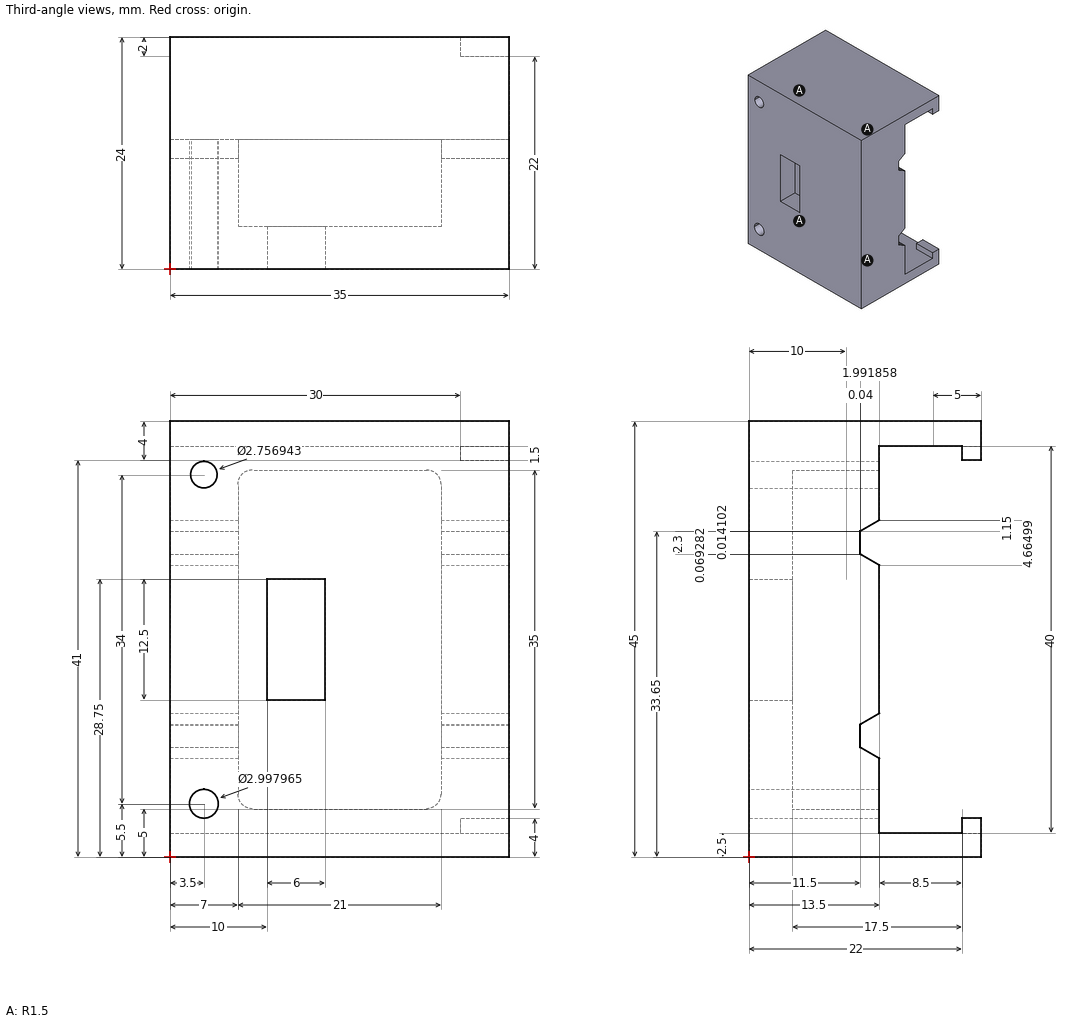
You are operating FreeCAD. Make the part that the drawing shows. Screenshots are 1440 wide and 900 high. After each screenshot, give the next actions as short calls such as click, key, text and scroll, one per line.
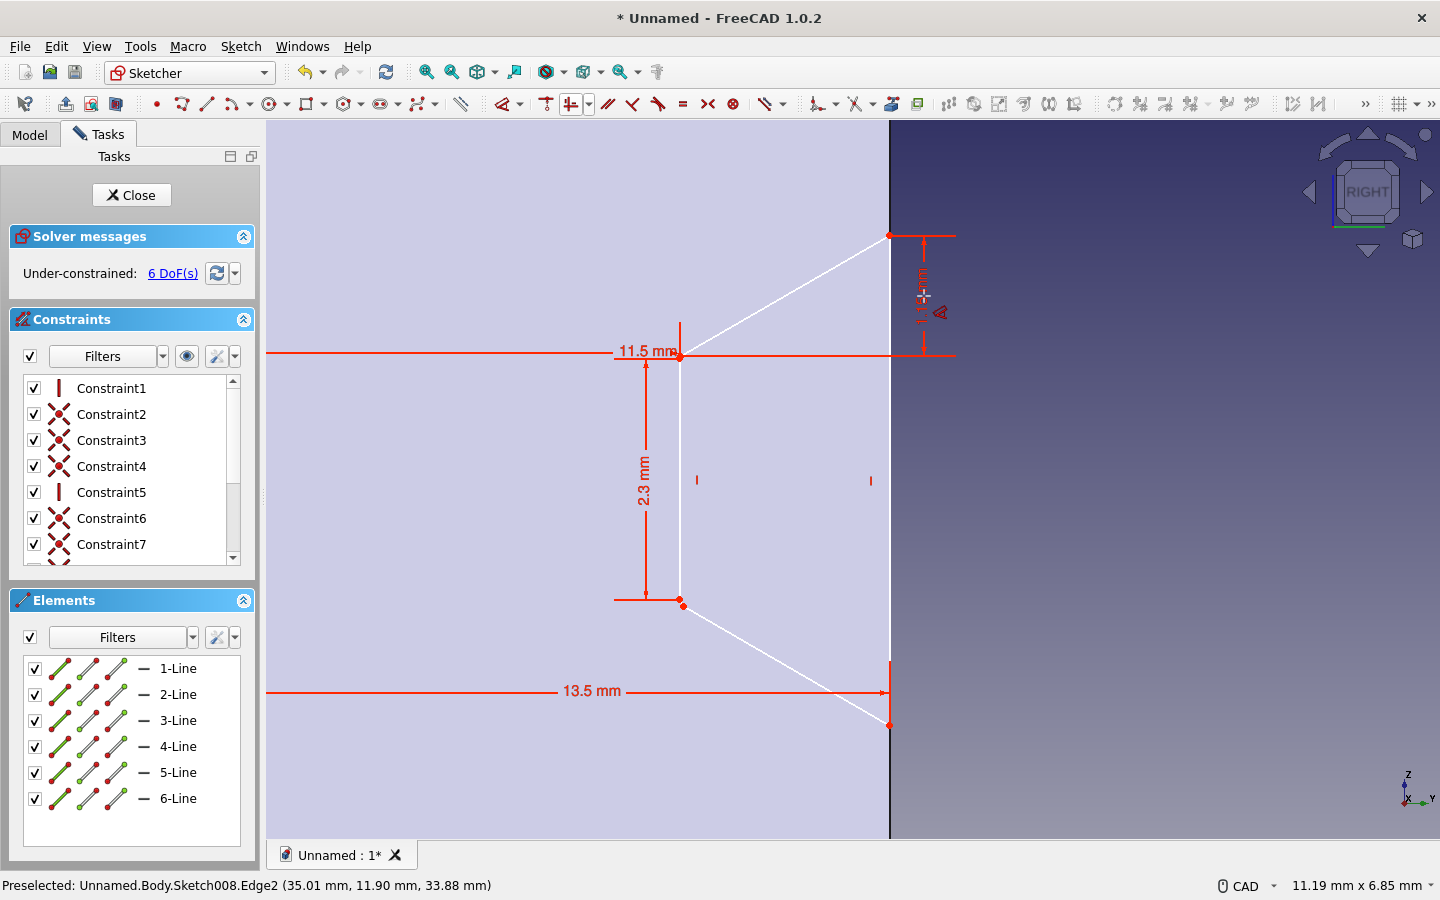
scroll(682, 603, up, 12)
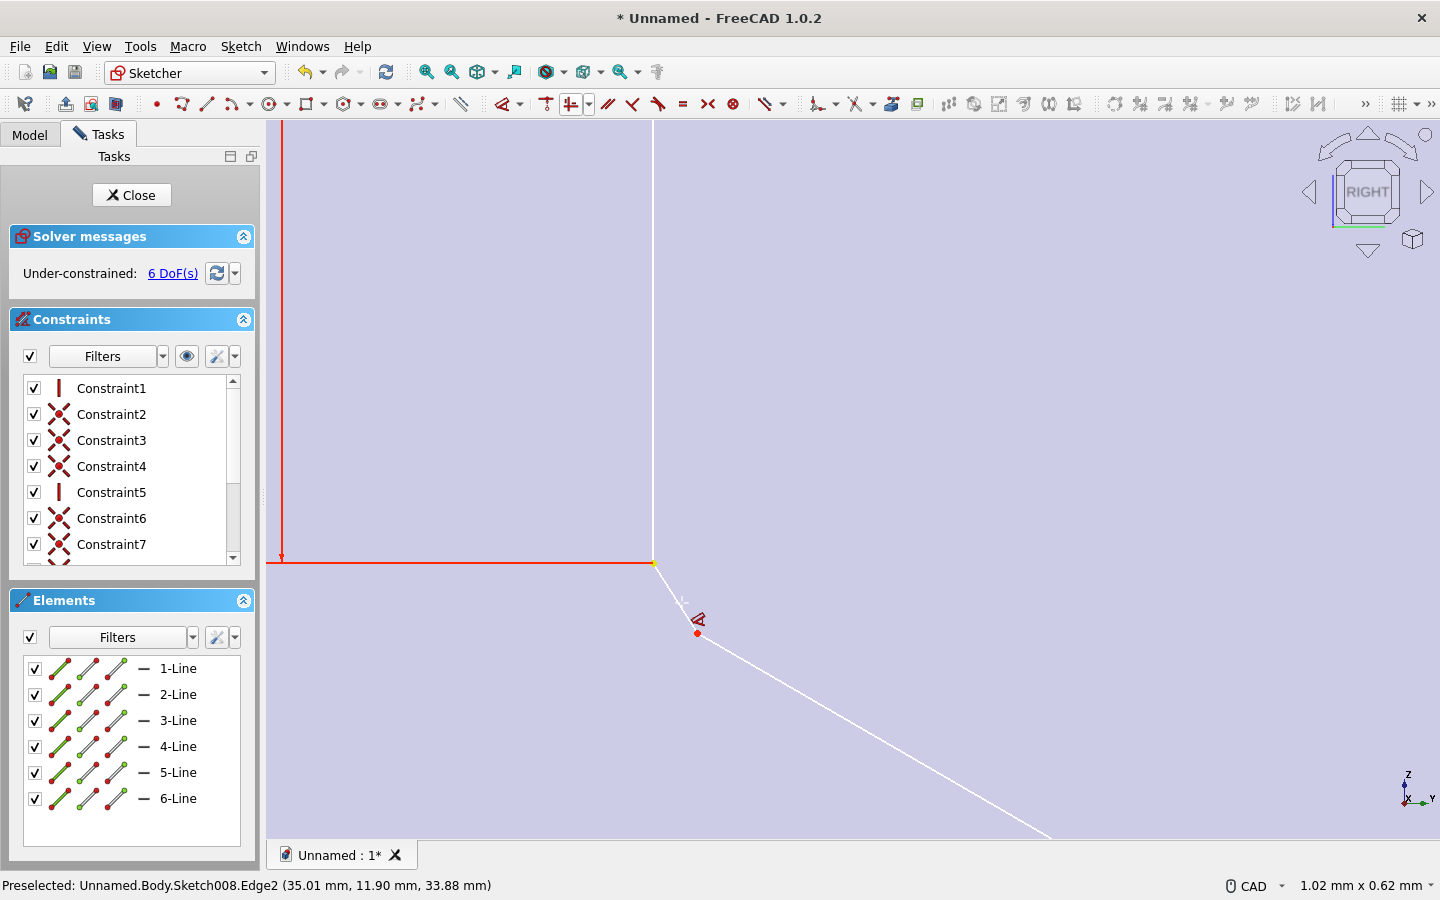
click(675, 598)
click(675, 667)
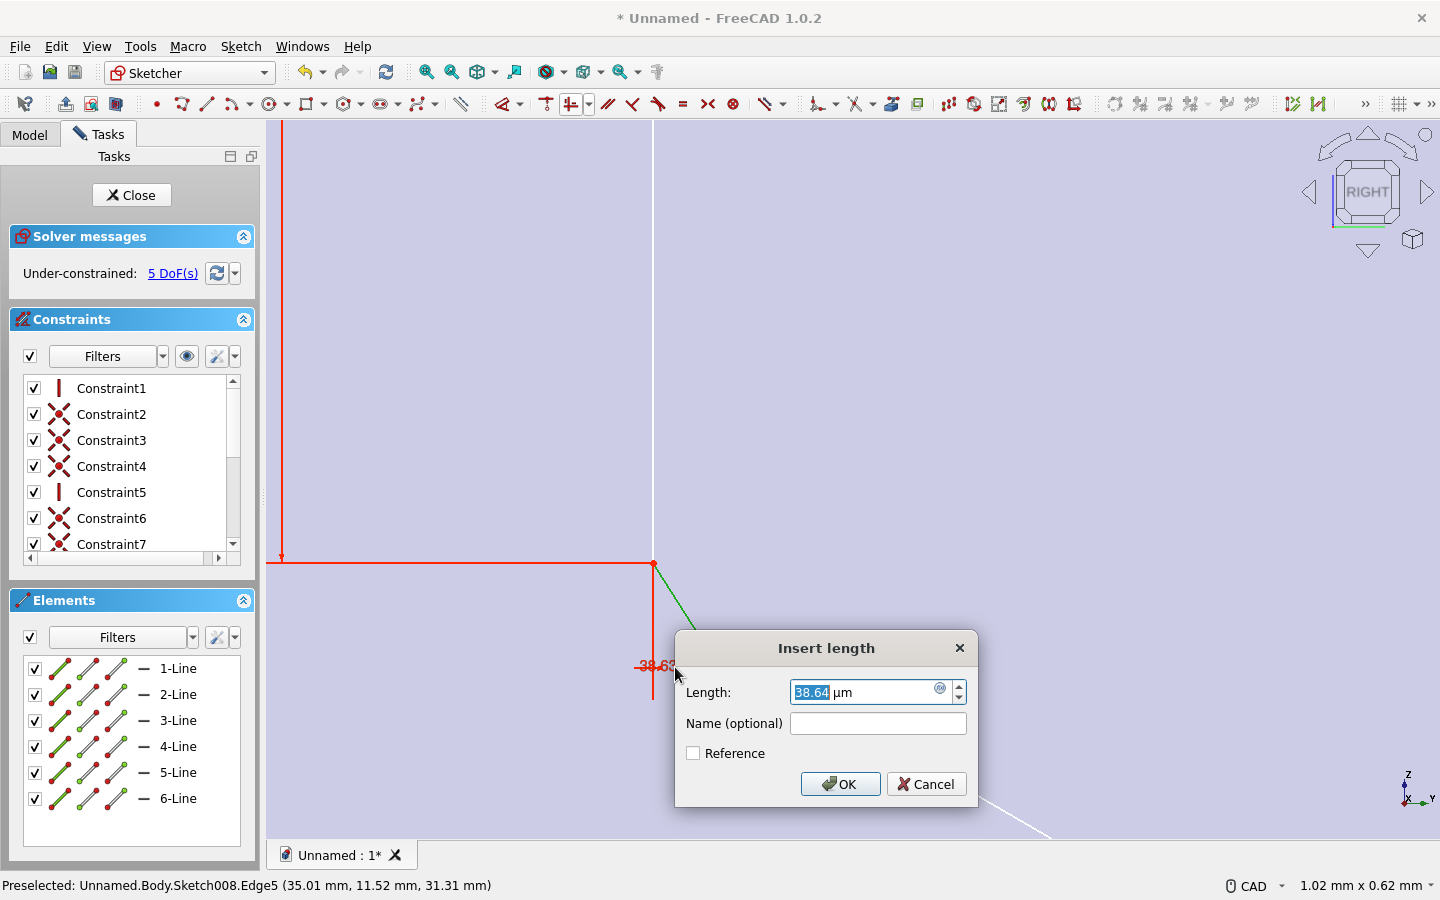
key(ctrl+a)
text(0.04 mm)
key(Return)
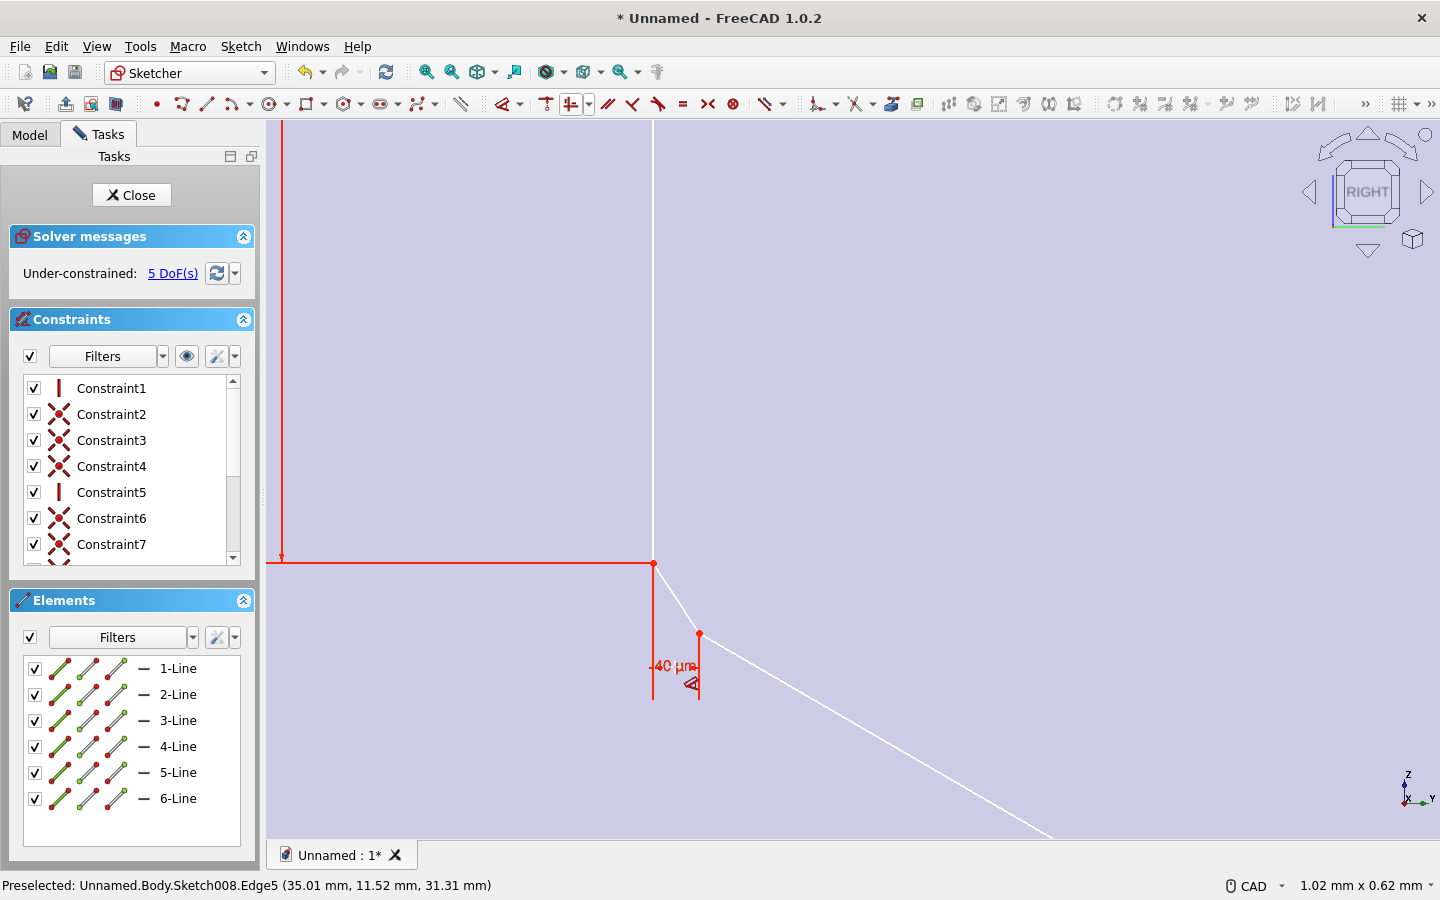
scroll(682, 603, down, 12)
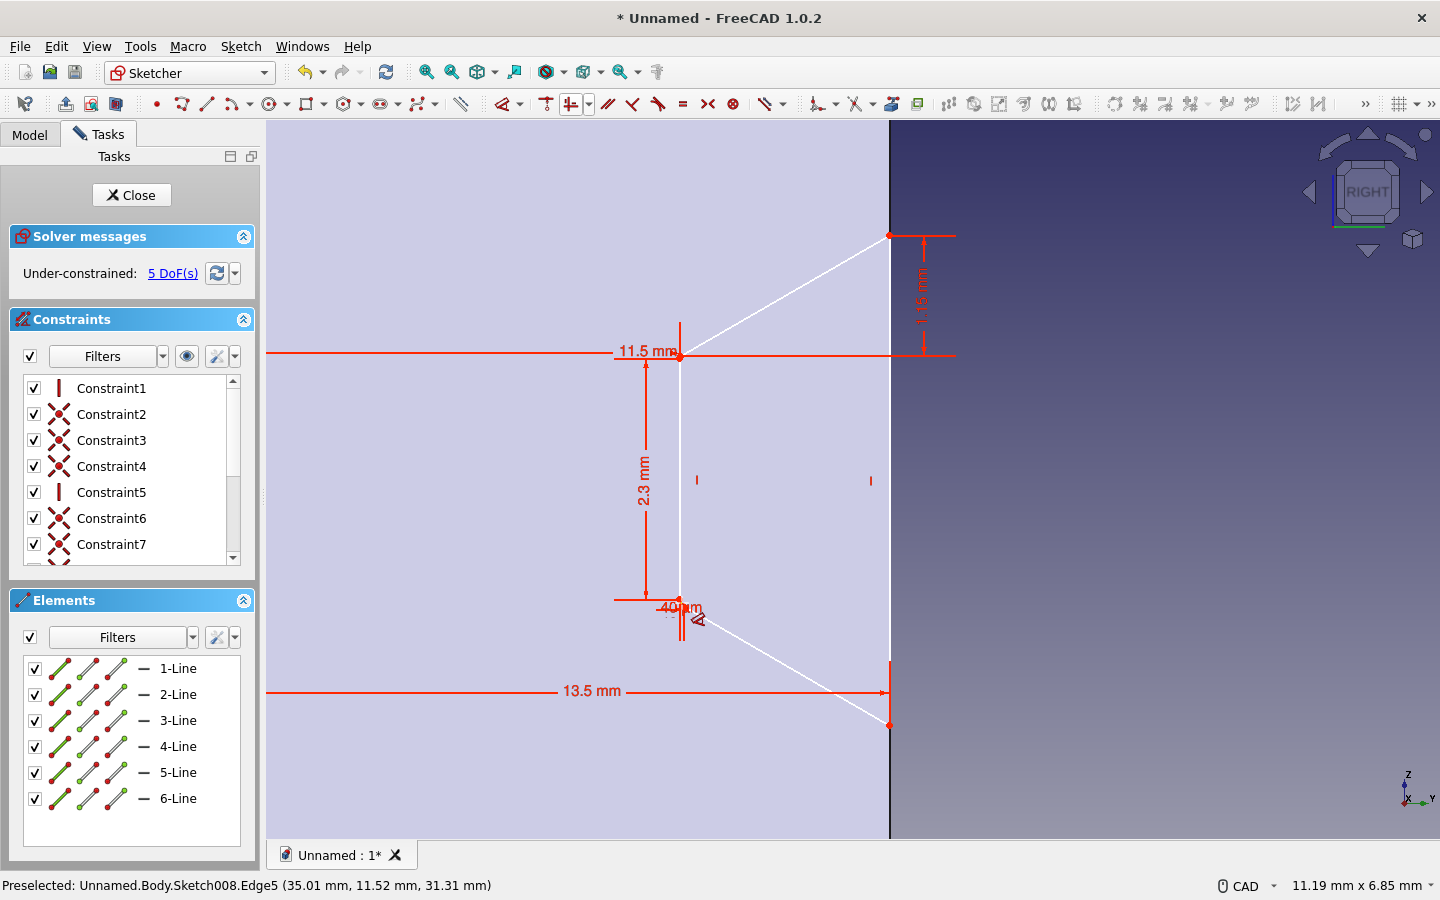
scroll(680, 359, up, 8)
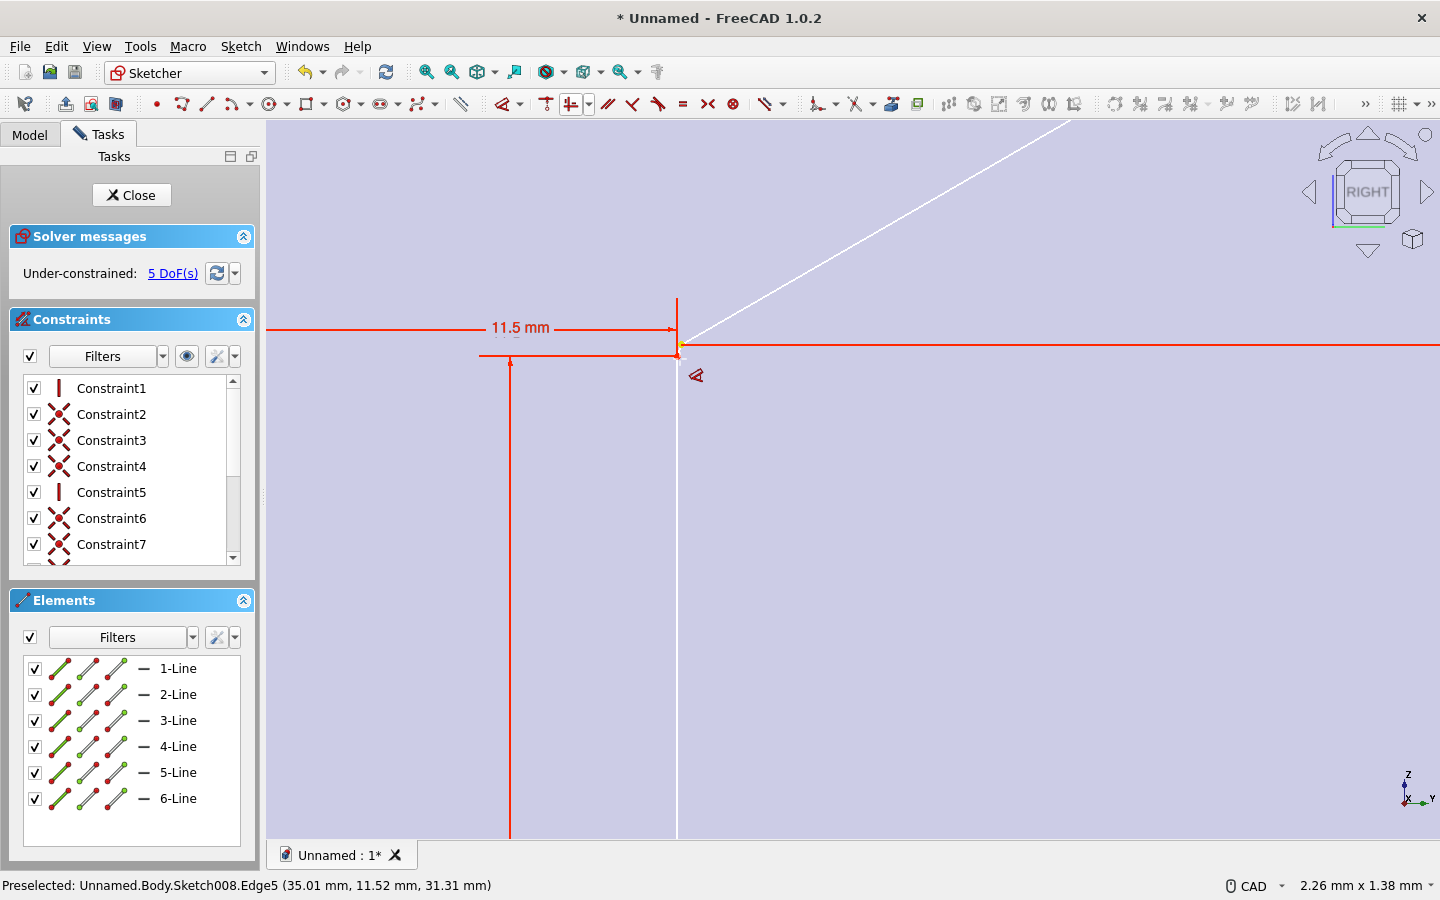
click(677, 356)
click(711, 584)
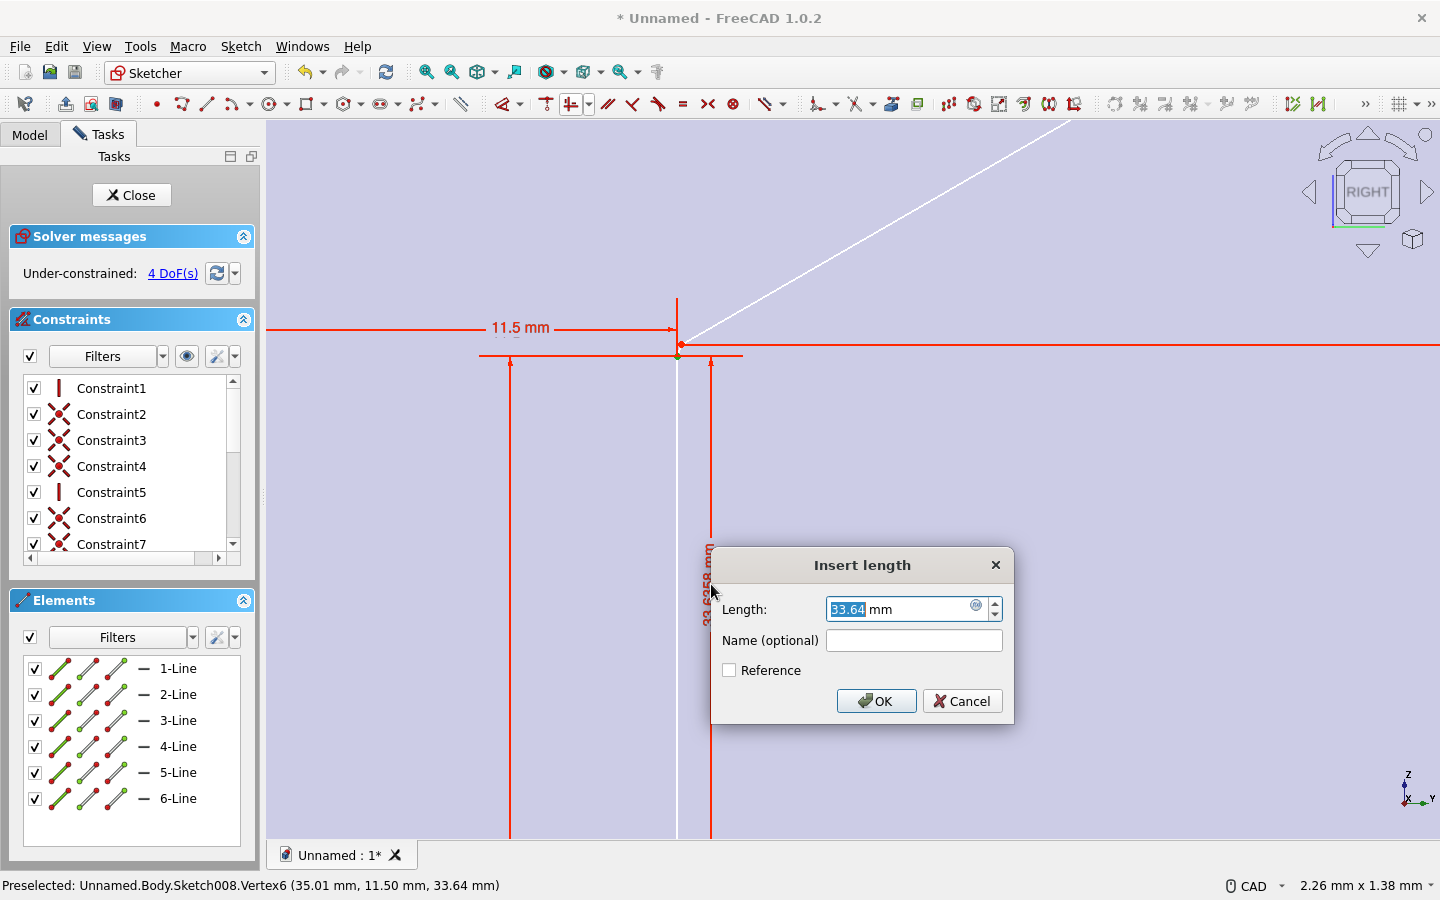
text(33.65)
key(Return)